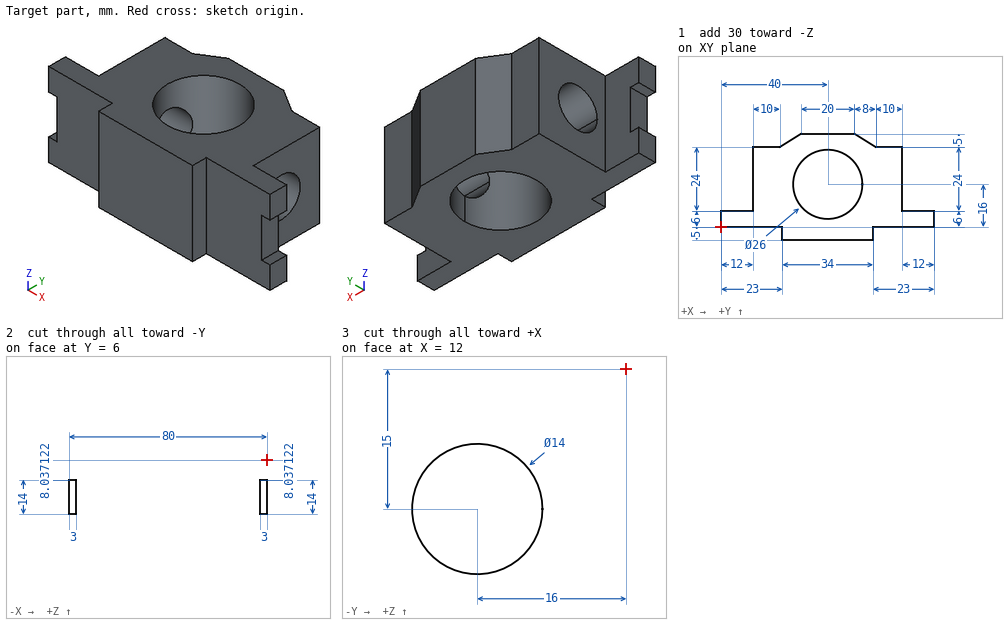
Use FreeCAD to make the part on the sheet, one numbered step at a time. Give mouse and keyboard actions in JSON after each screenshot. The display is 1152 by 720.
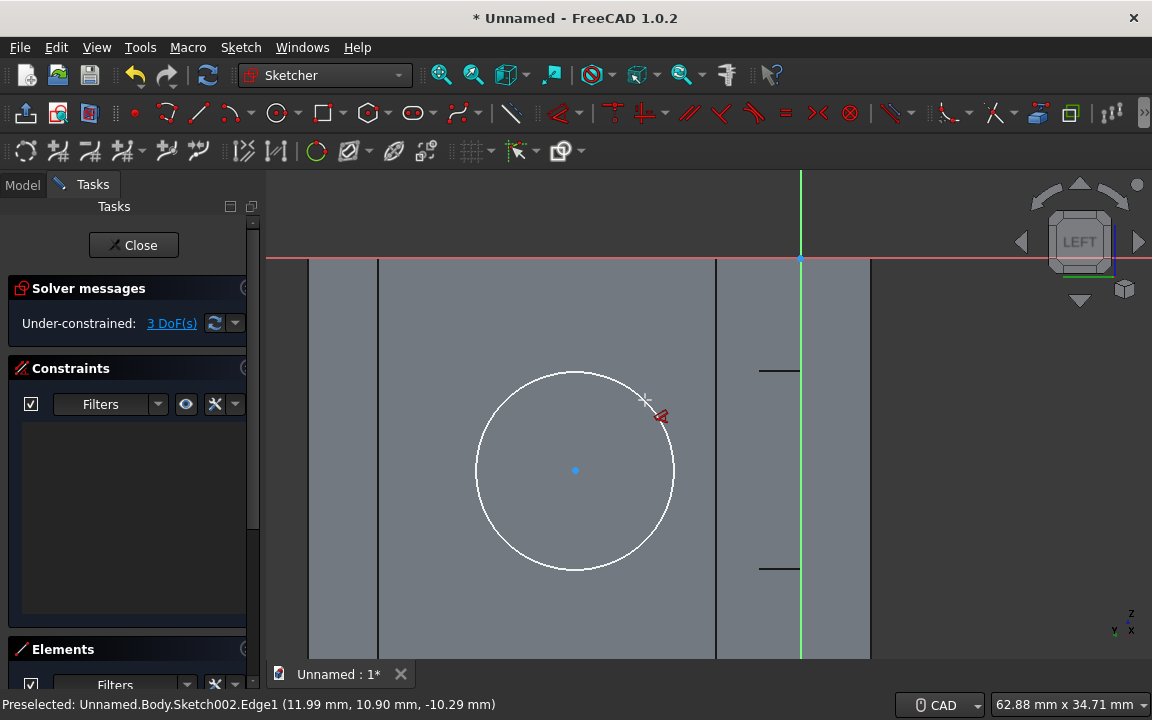
{"action": "left_click", "coordinate": [645, 401]}
{"action": "left_click", "coordinate": [668, 378]}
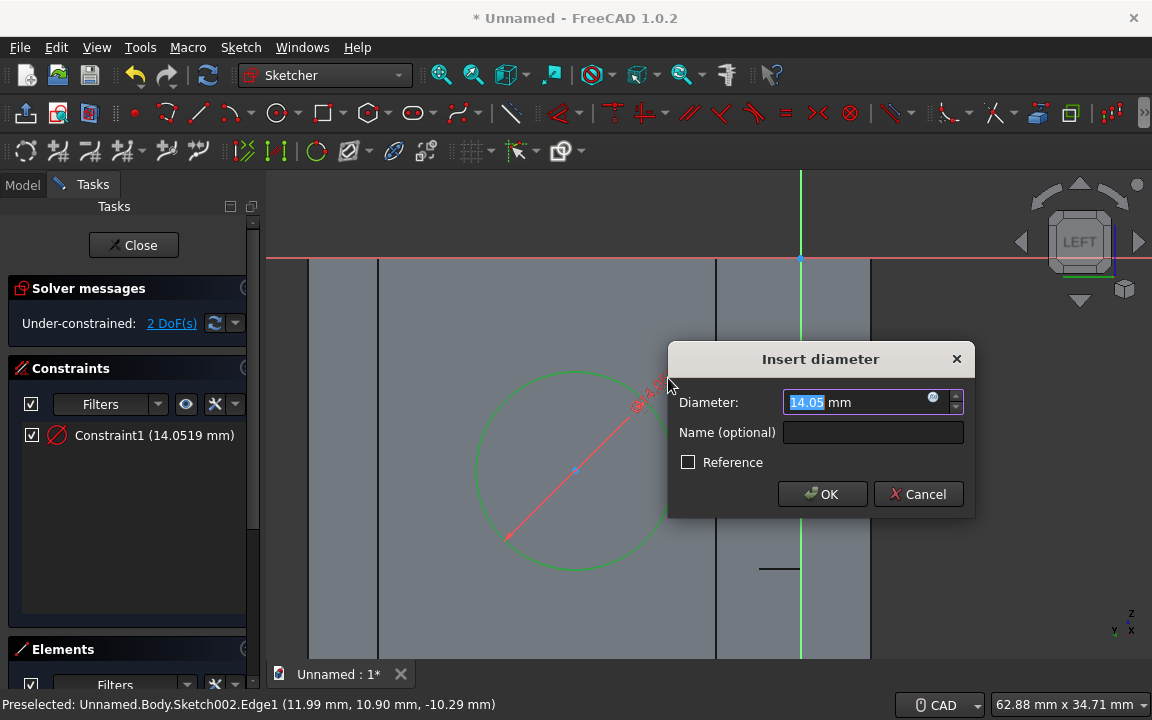
{"action": "type", "text": "14"}
{"action": "key", "text": "Return"}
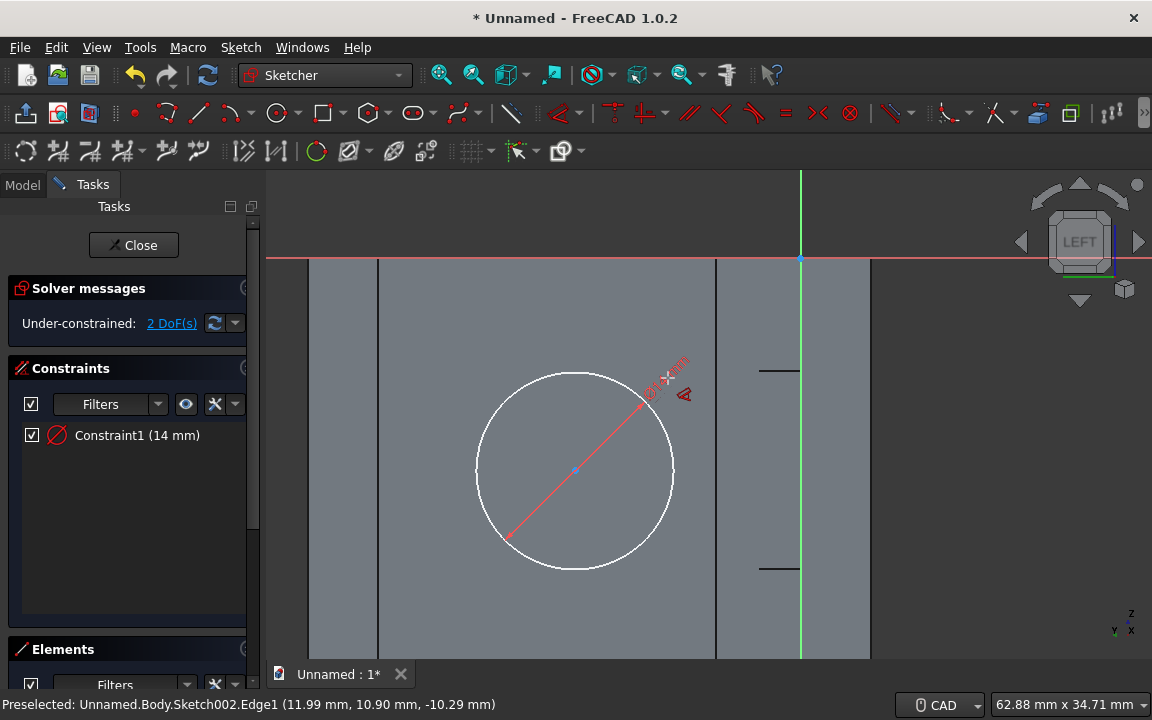
{"action": "left_click", "coordinate": [575, 471]}
{"action": "left_click", "coordinate": [688, 224]}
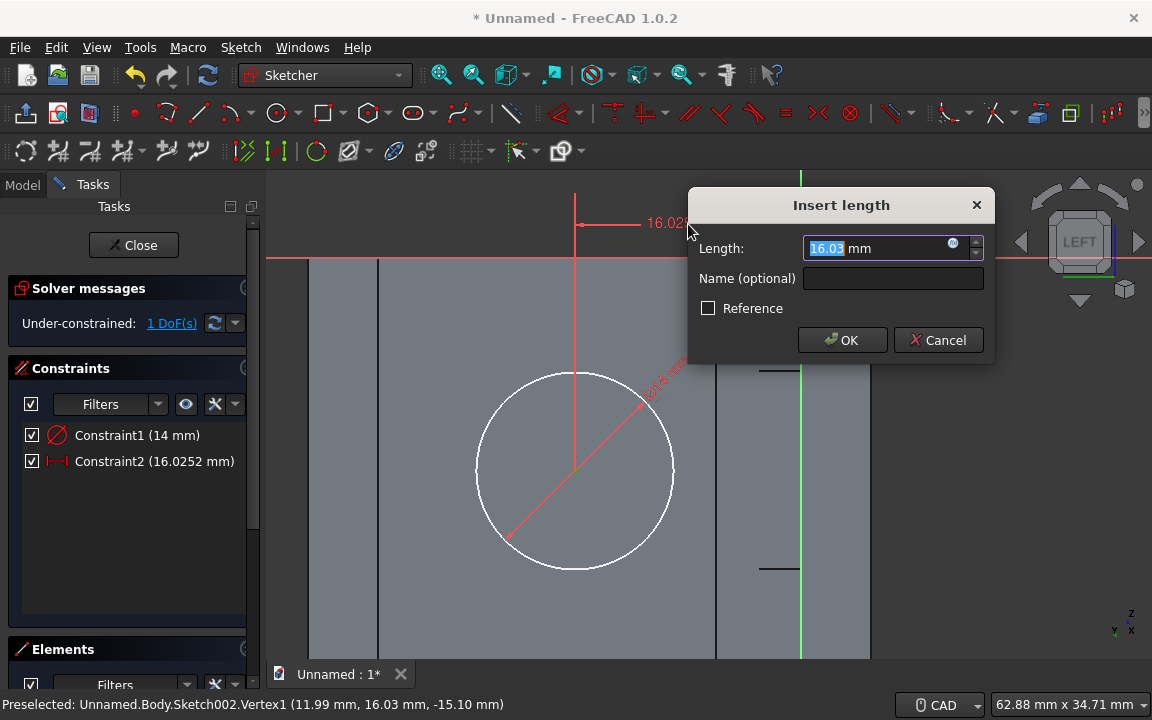
{"action": "type", "text": "16"}
{"action": "key", "text": "Return"}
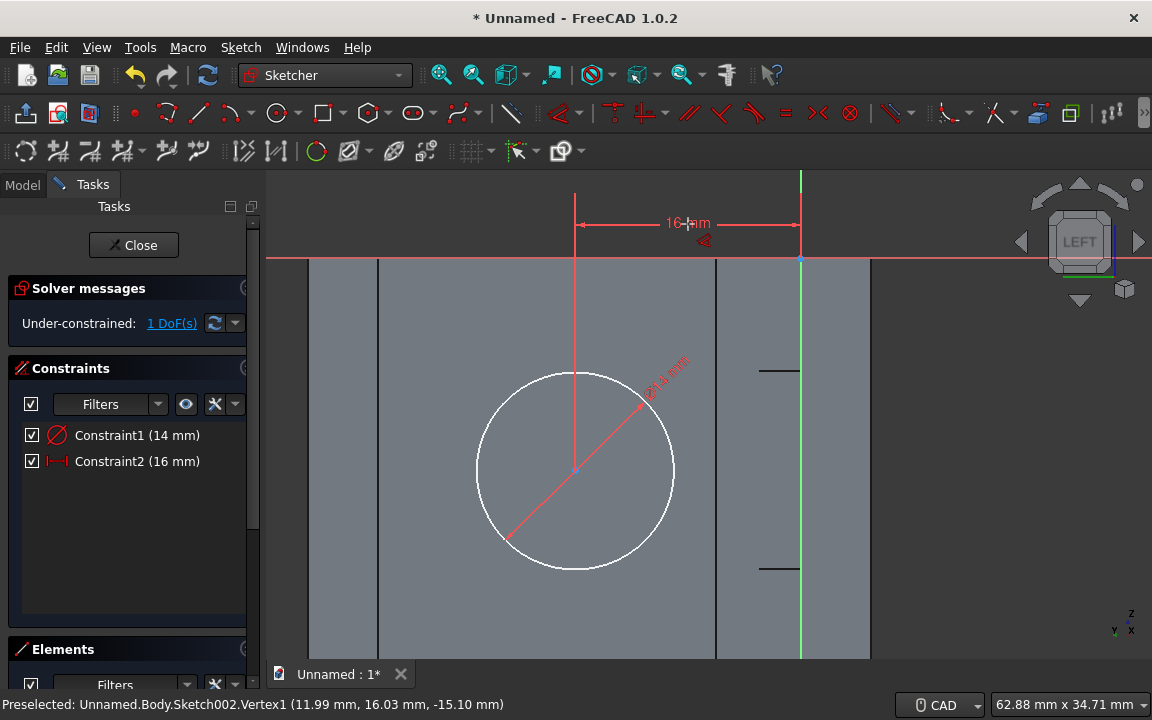
{"action": "left_click", "coordinate": [575, 471]}
{"action": "left_click", "coordinate": [835, 365]}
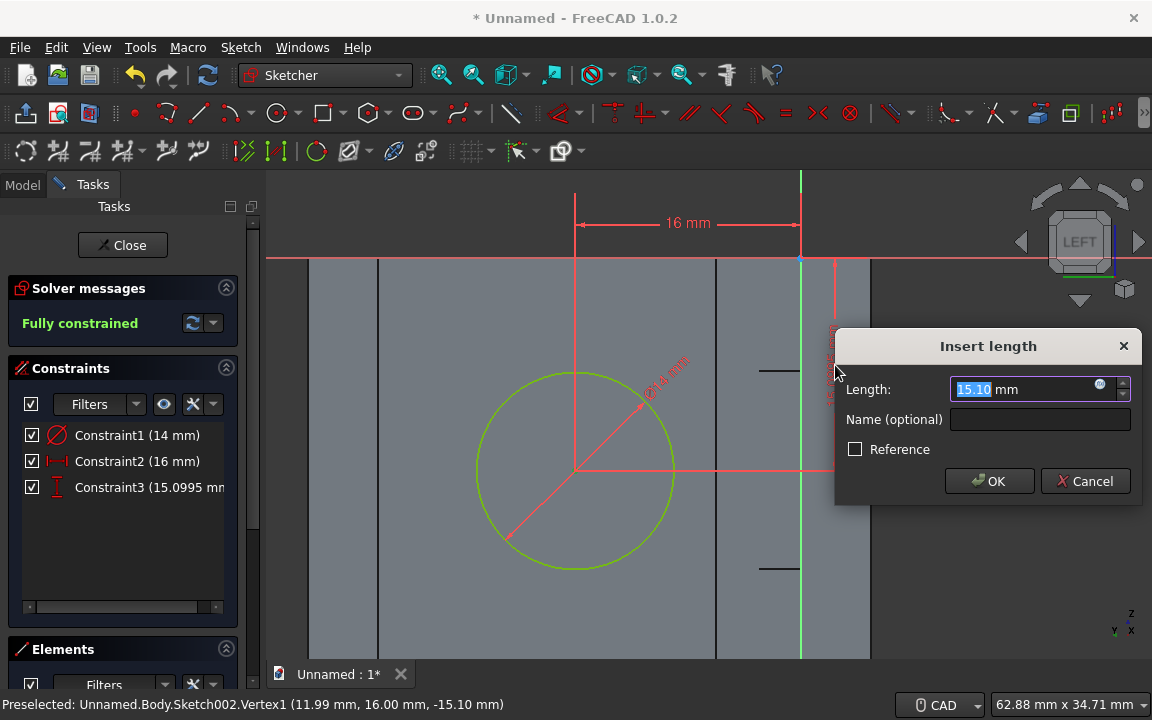
{"action": "type", "text": "15"}
{"action": "key", "text": "Return"}
{"action": "key", "text": "Escape"}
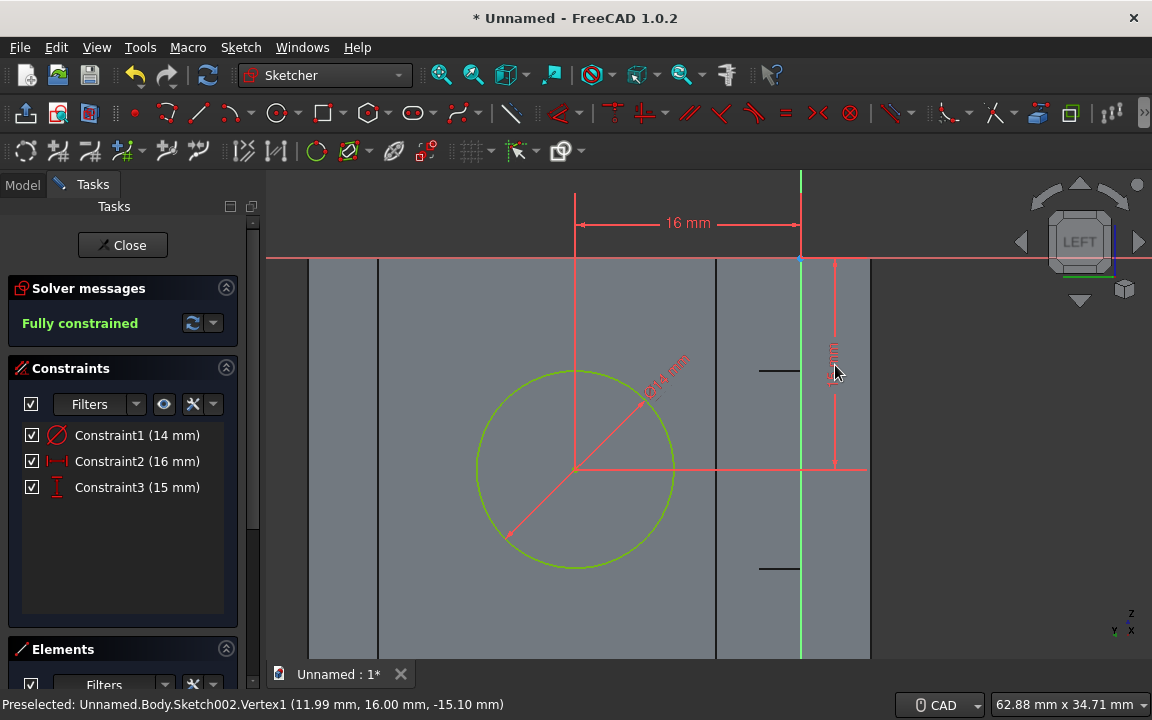
{"action": "left_click", "coordinate": [123, 245]}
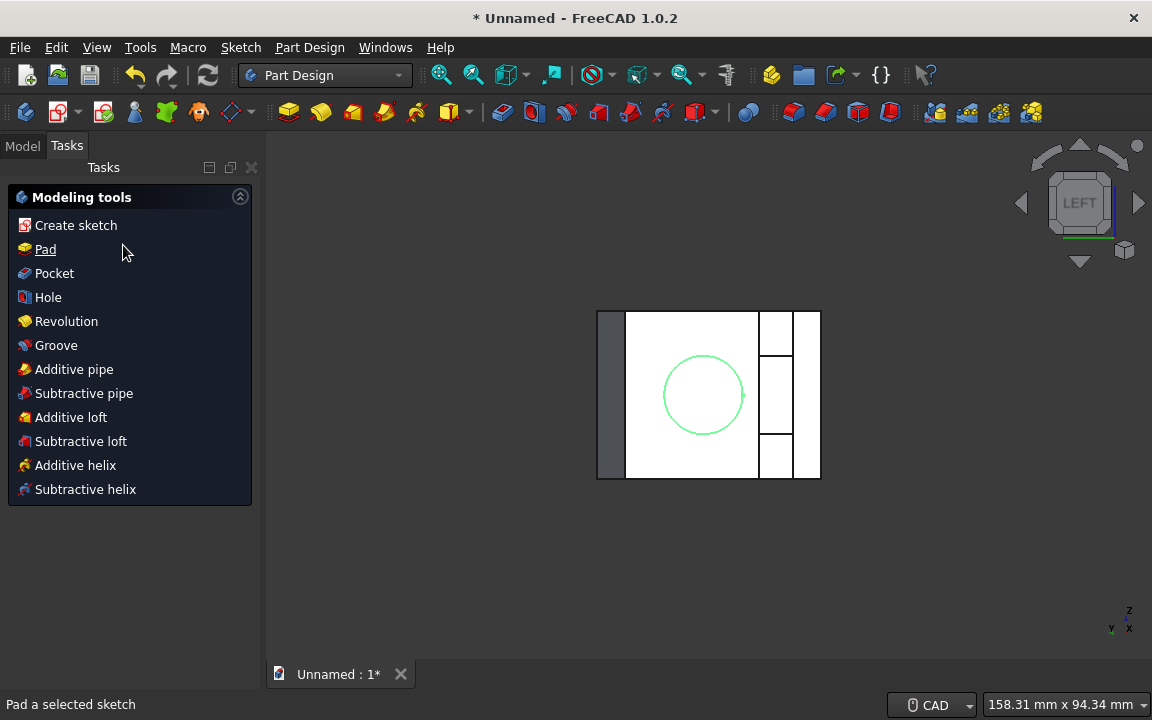
{"action": "left_click", "coordinate": [504, 112]}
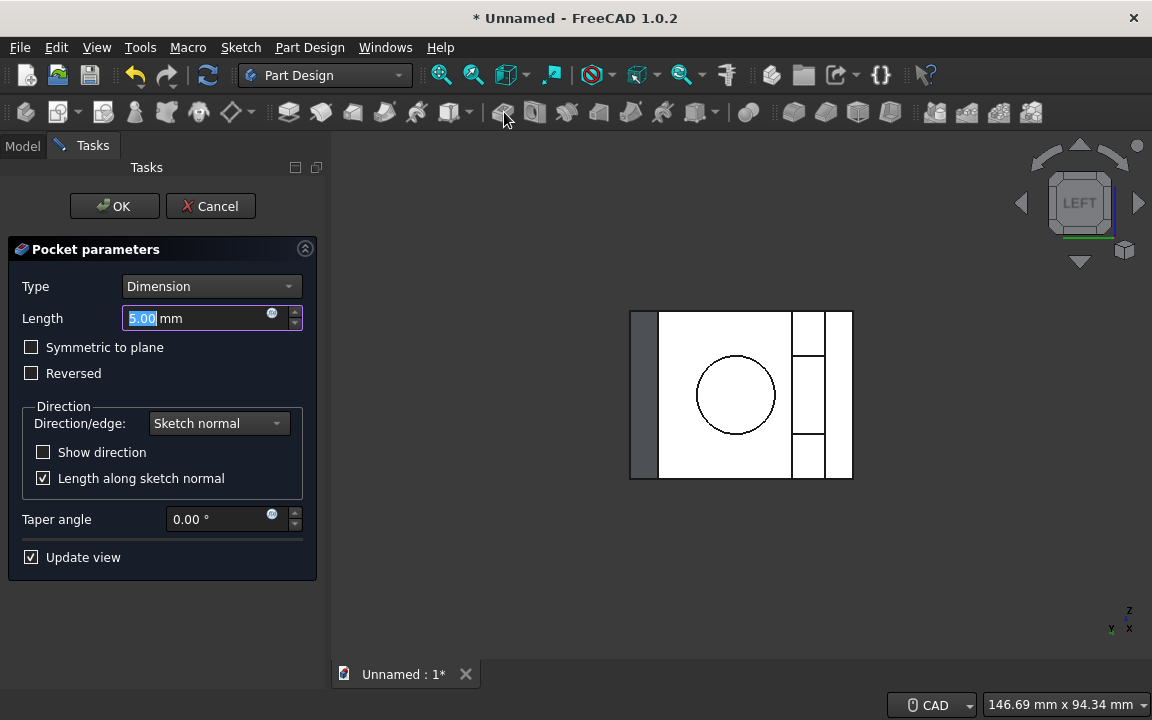
{"action": "left_click", "coordinate": [212, 286]}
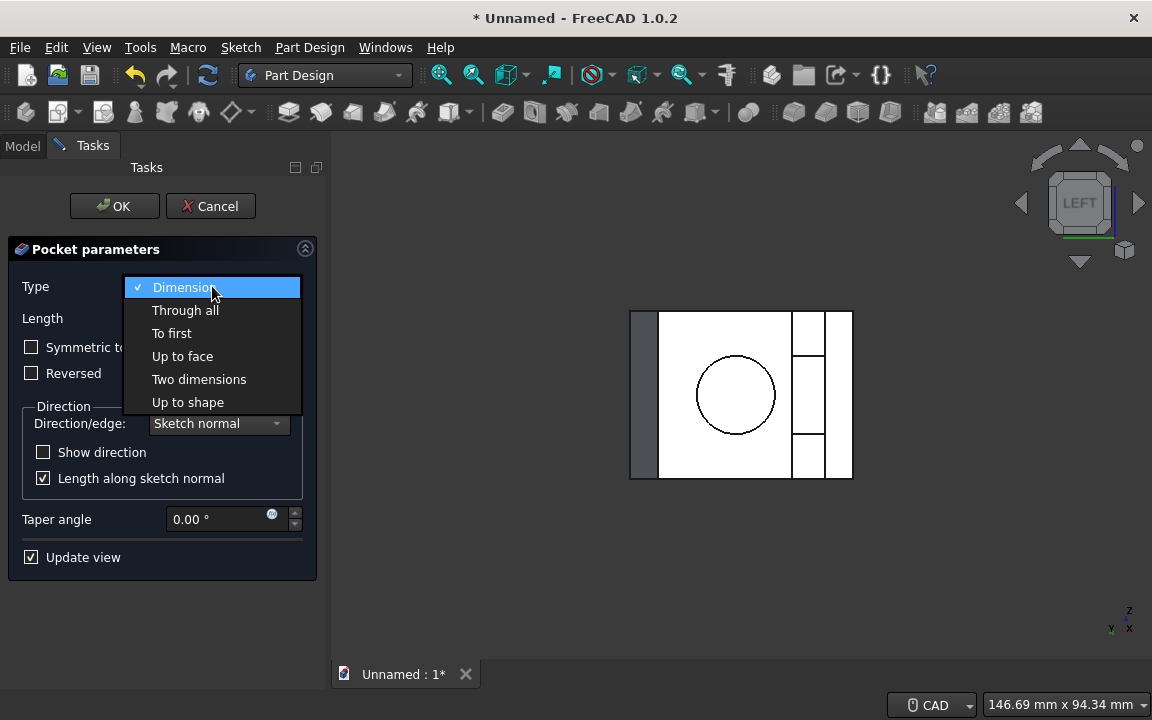
{"action": "left_click", "coordinate": [212, 310]}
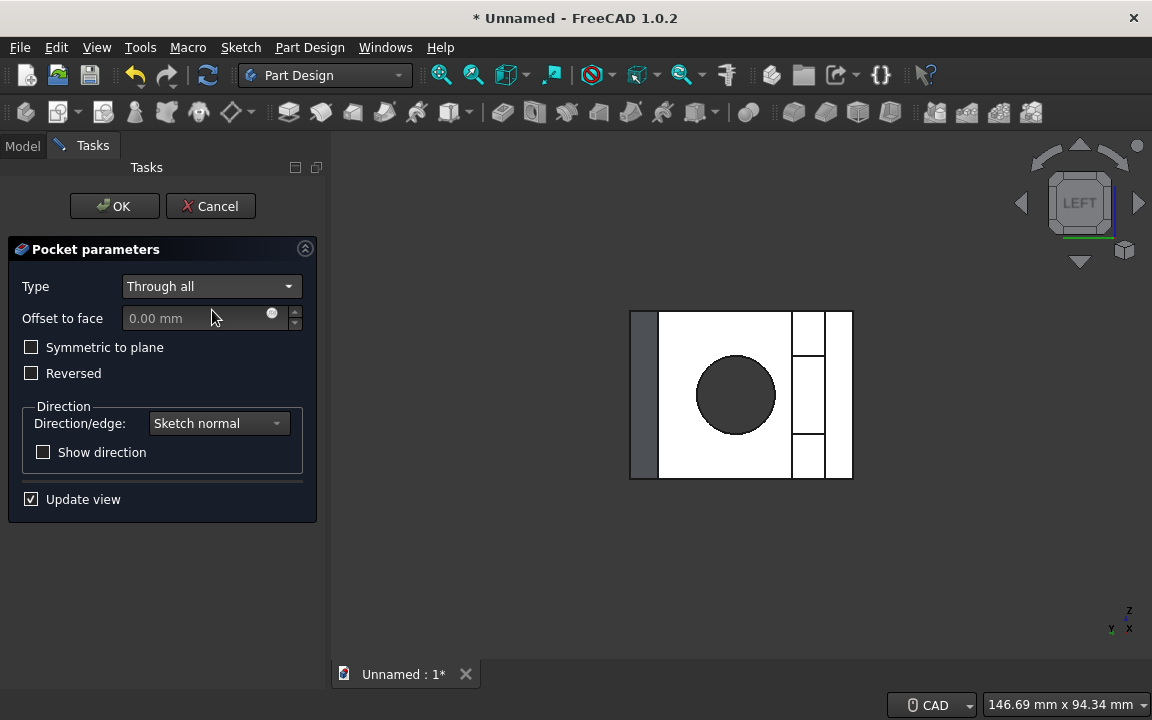
{"action": "left_click", "coordinate": [115, 206]}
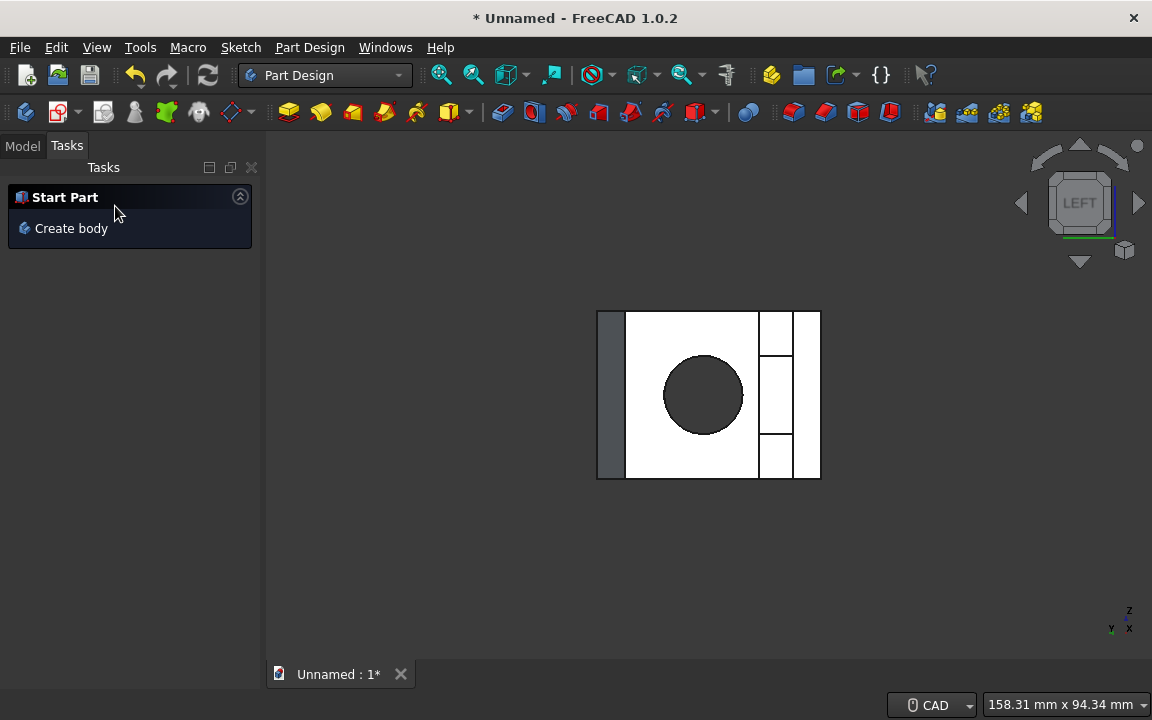
{"action": "key", "text": "0"}